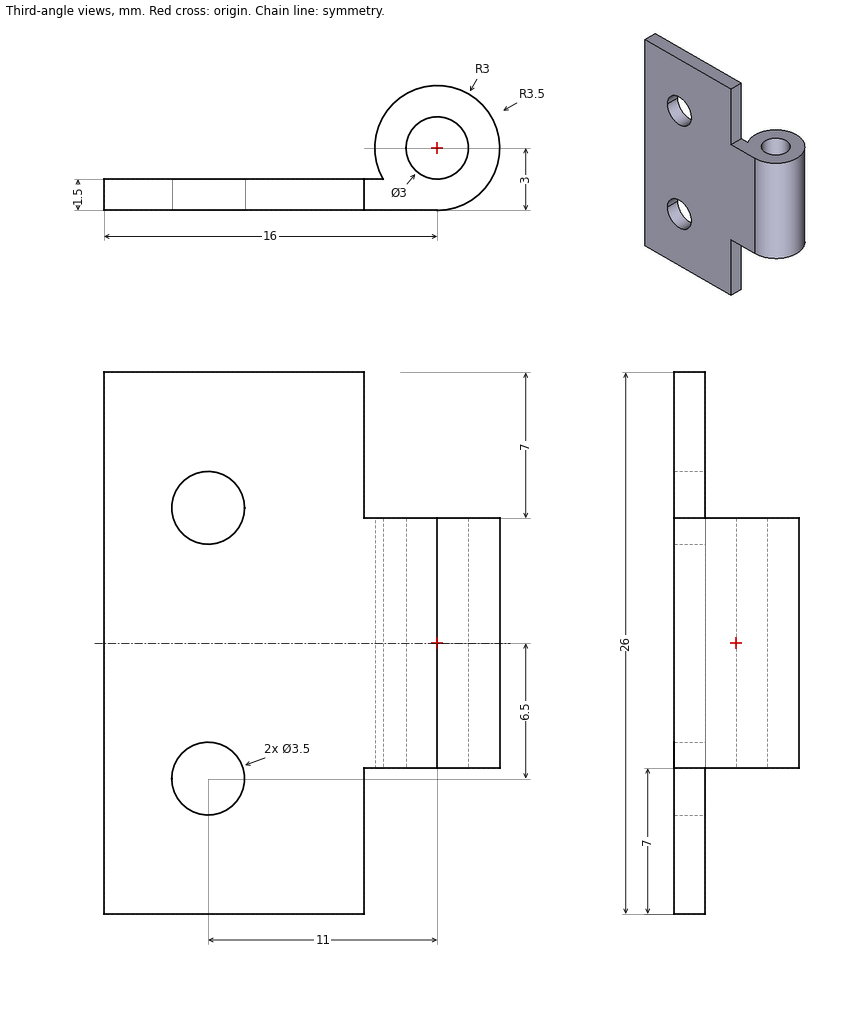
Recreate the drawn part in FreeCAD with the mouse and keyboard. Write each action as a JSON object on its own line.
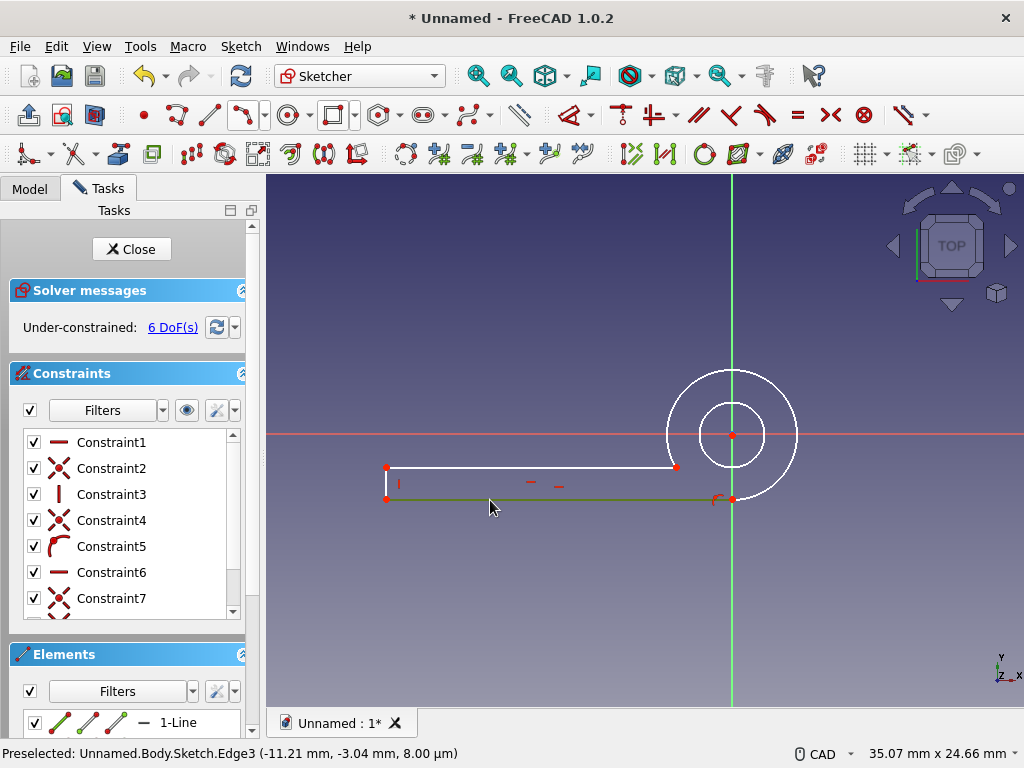
{"action": "left_click", "coordinate": [797, 435]}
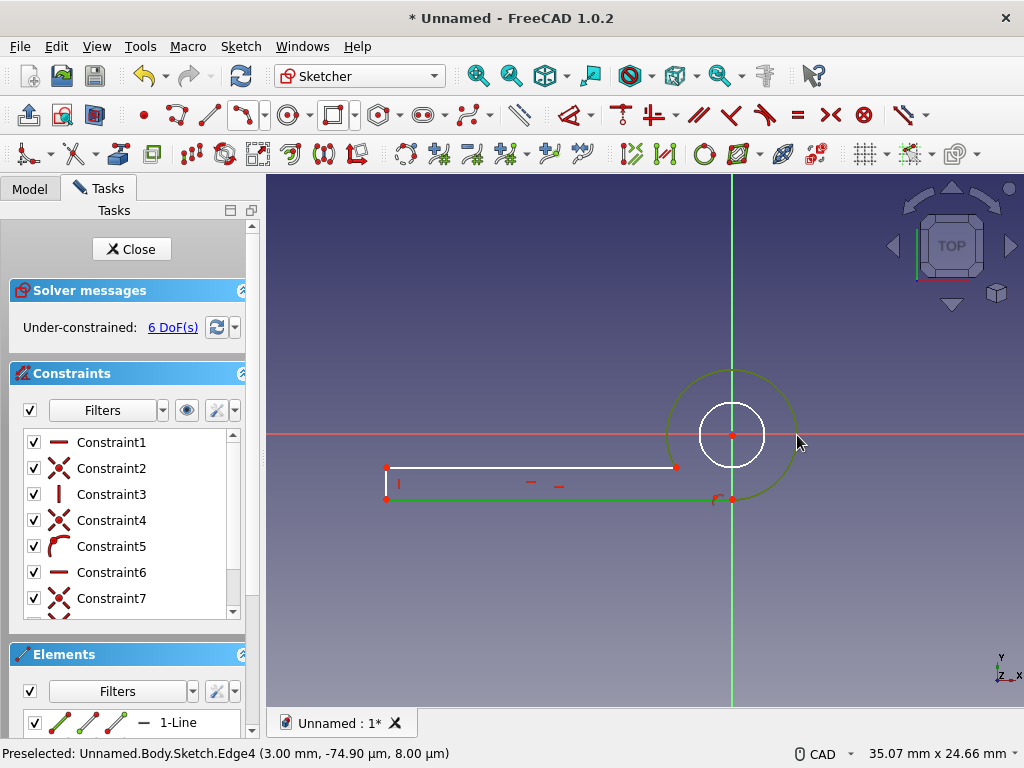
{"action": "left_click", "coordinate": [765, 116]}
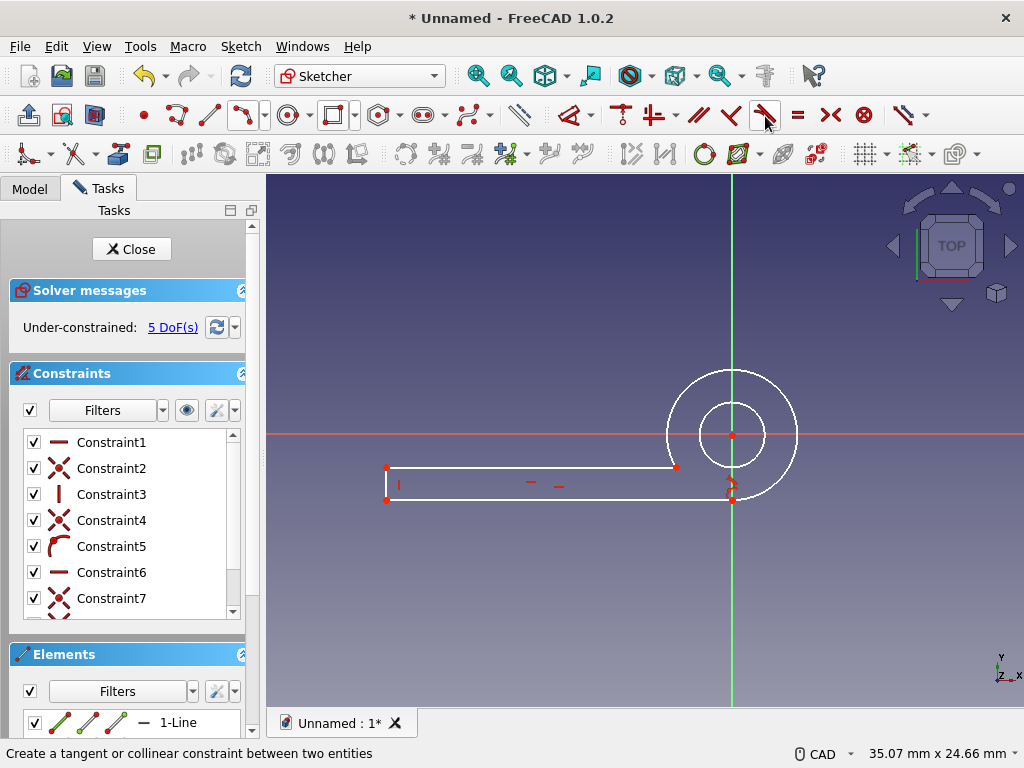
{"action": "left_click", "coordinate": [732, 435]}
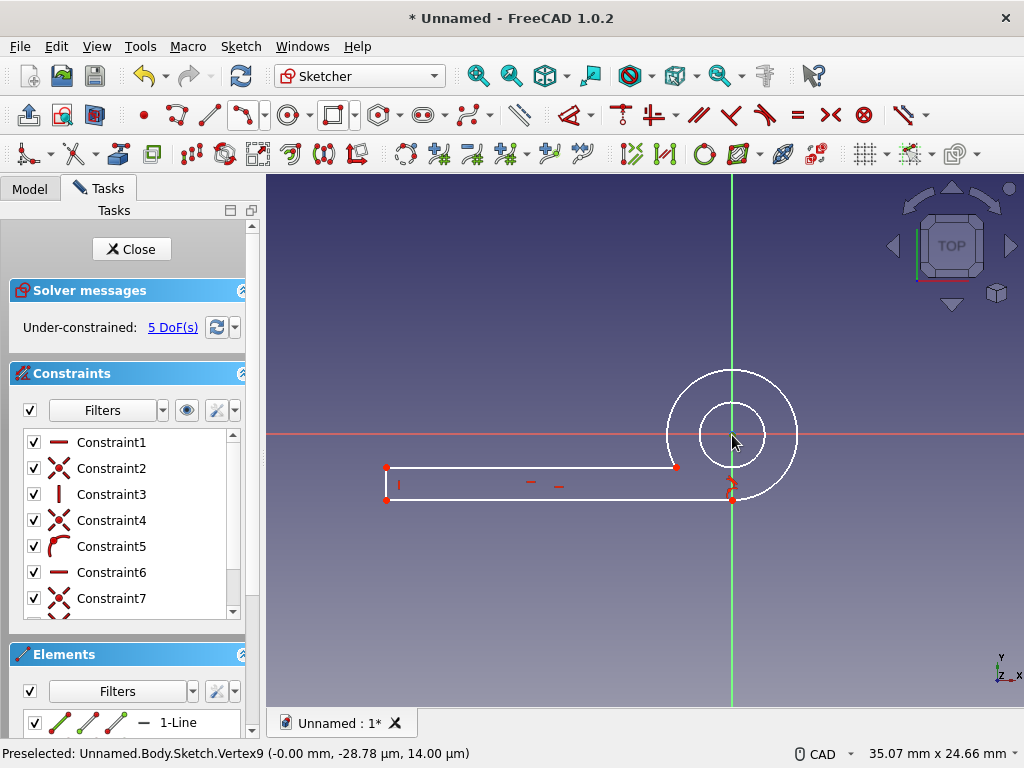
{"action": "left_click", "coordinate": [334, 434]}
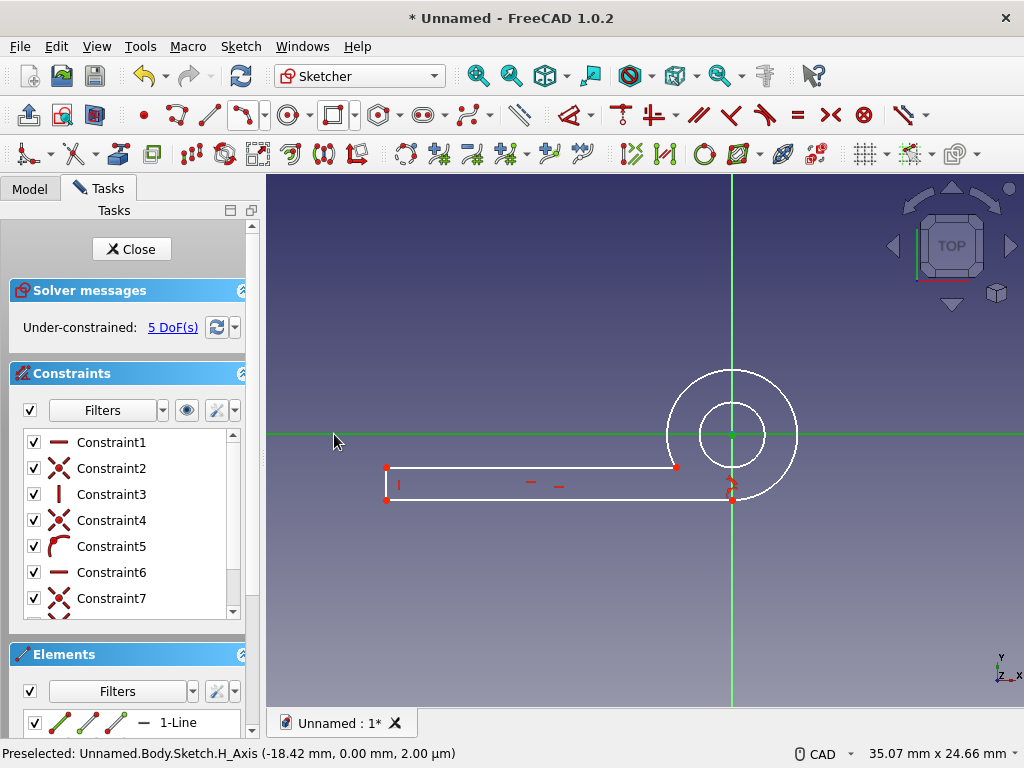
{"action": "left_click", "coordinate": [621, 116]}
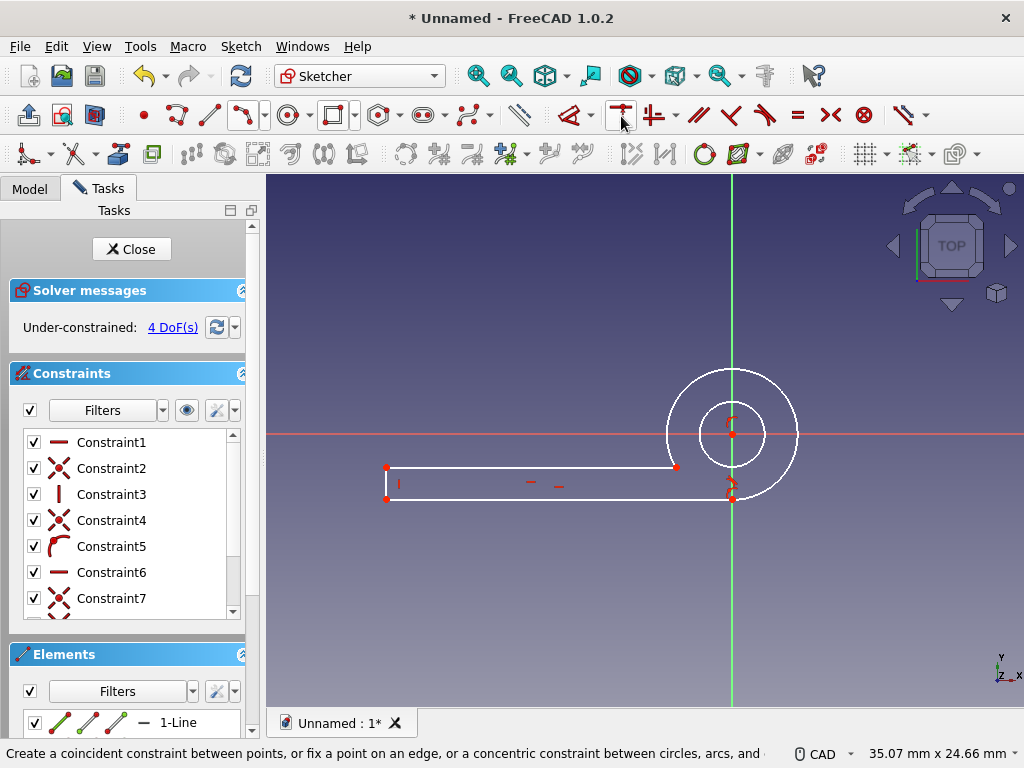
{"action": "left_click", "coordinate": [798, 434]}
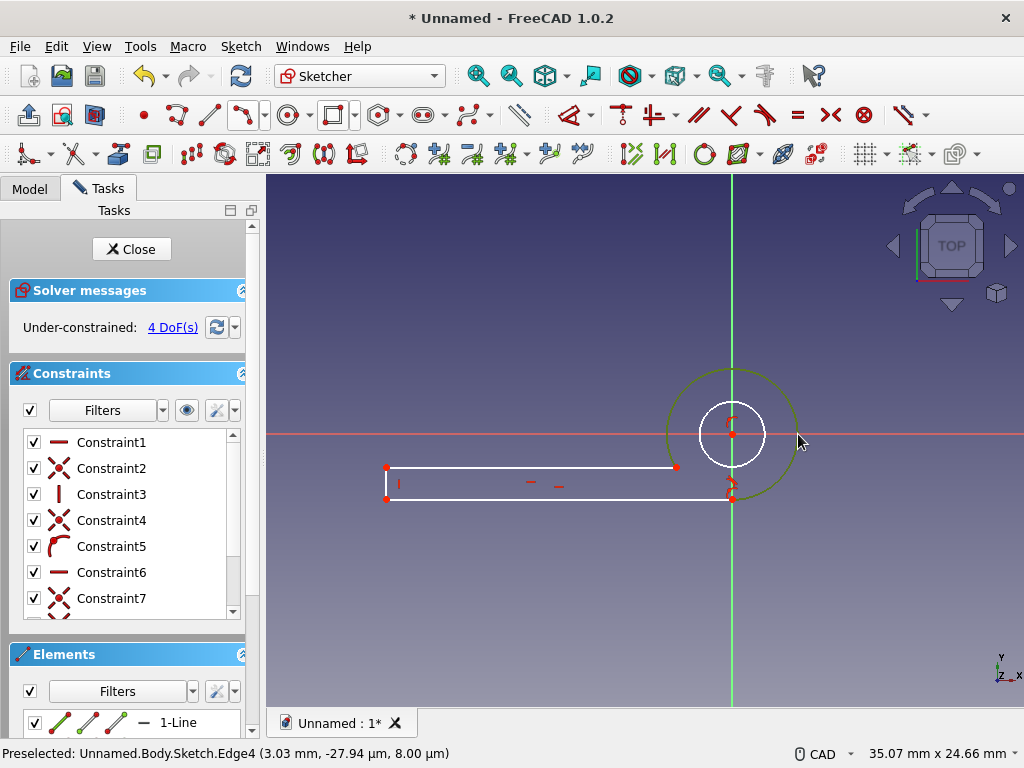
{"action": "key", "text": "k r"}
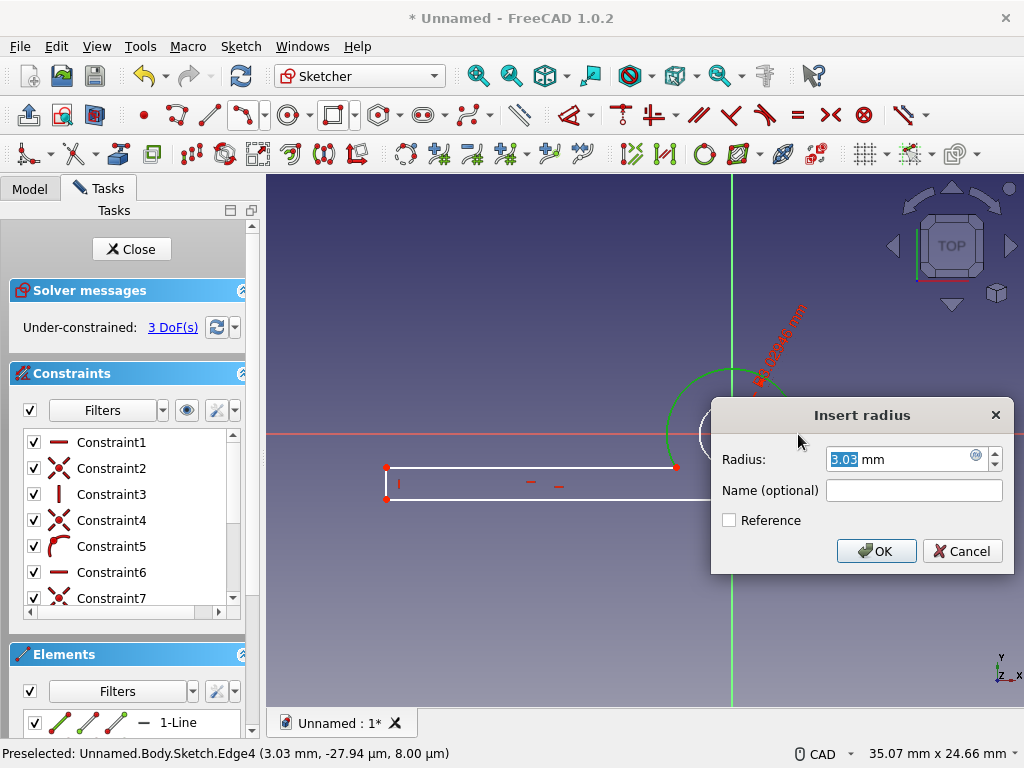
{"action": "type", "text": "3"}
{"action": "key", "text": "Return"}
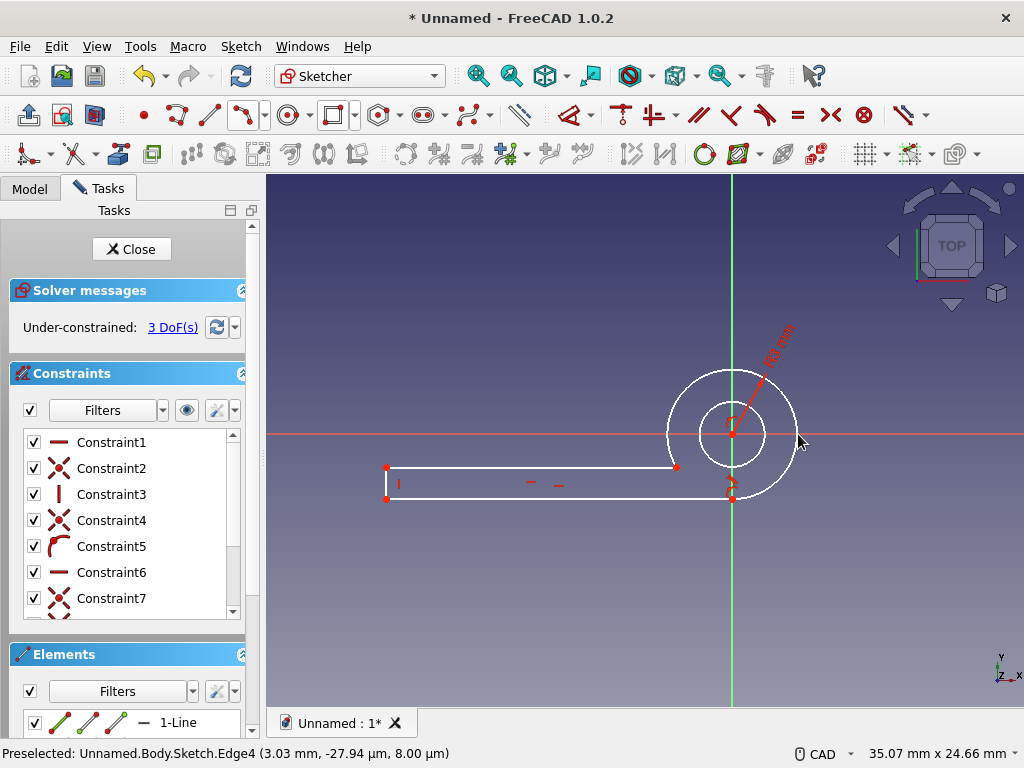
{"action": "left_click", "coordinate": [755, 411]}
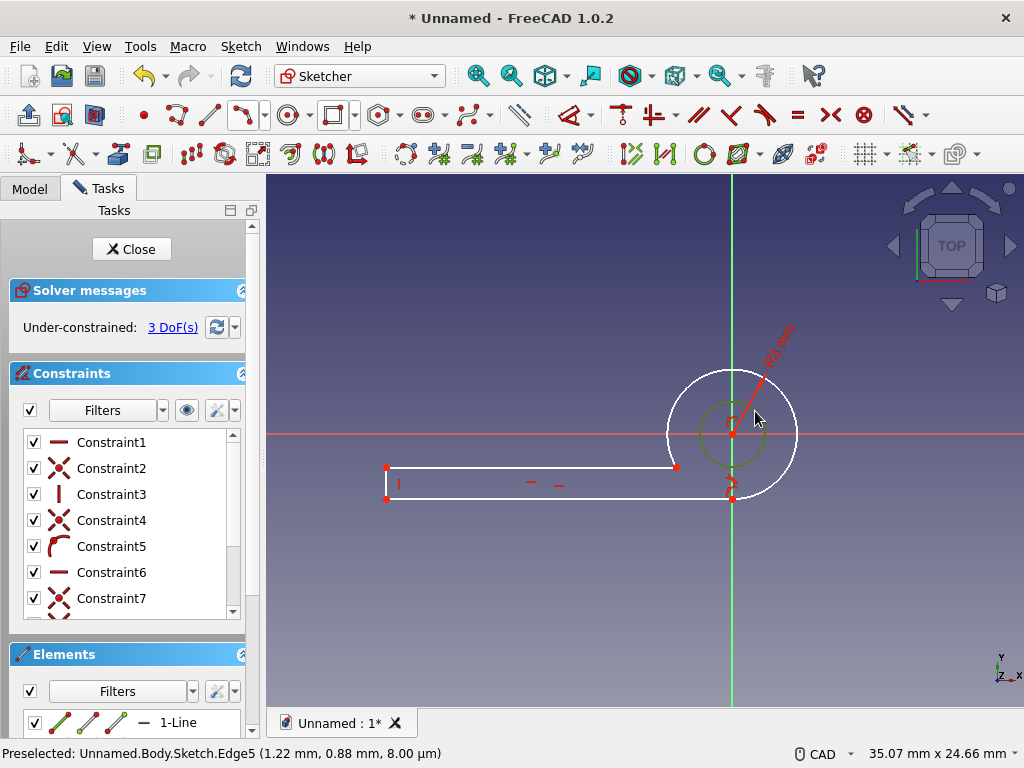
{"action": "left_click", "coordinate": [590, 116]}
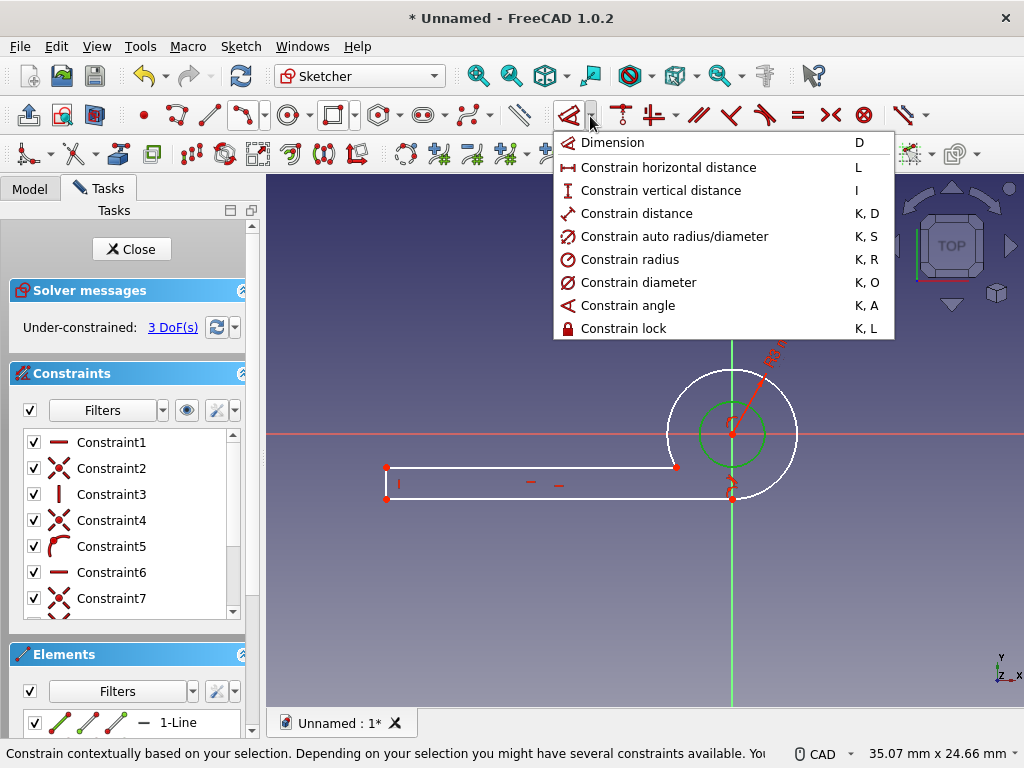
{"action": "left_click", "coordinate": [724, 282]}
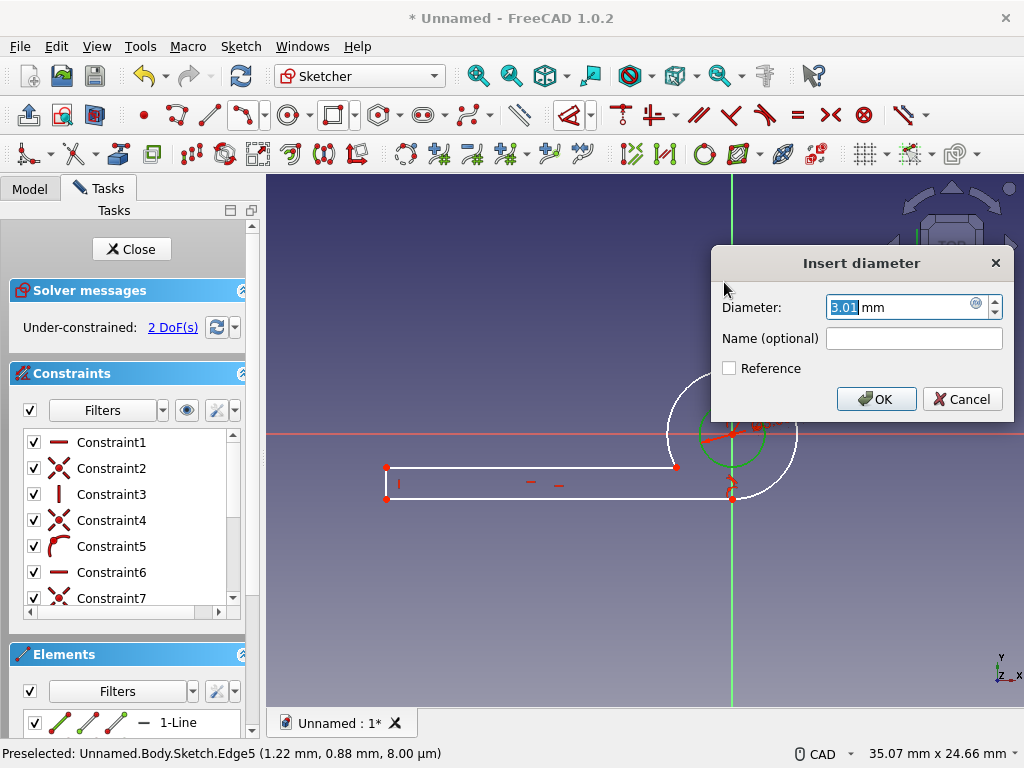
{"action": "type", "text": "3"}
{"action": "key", "text": "Return"}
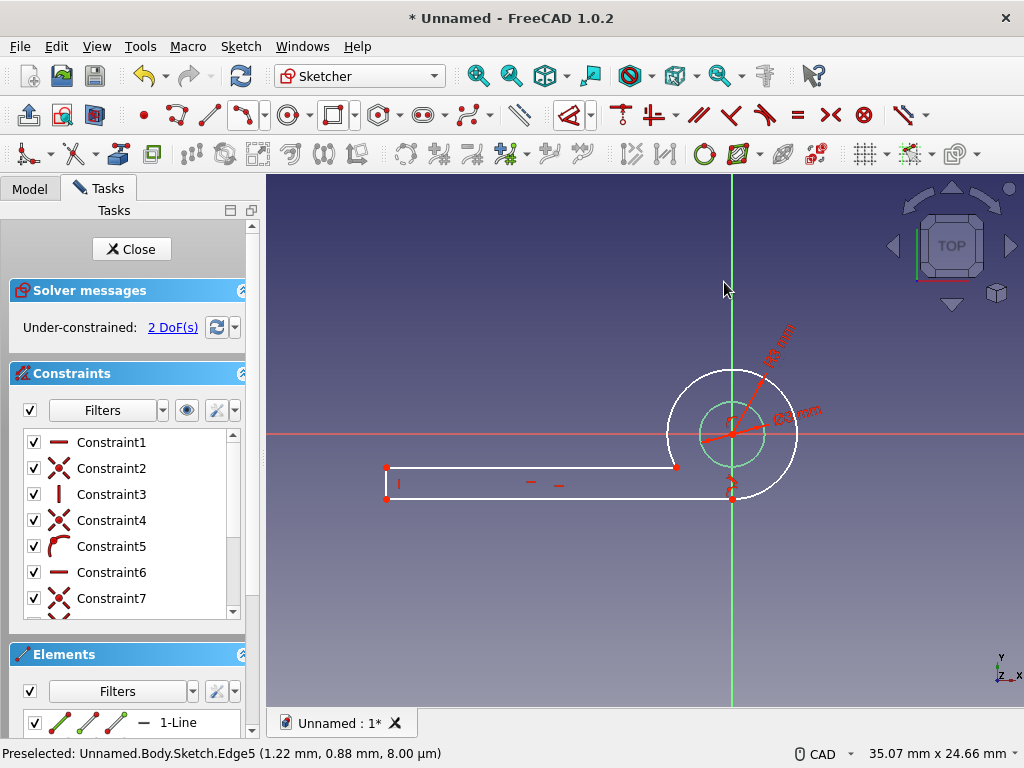
{"action": "left_click", "coordinate": [490, 499]}